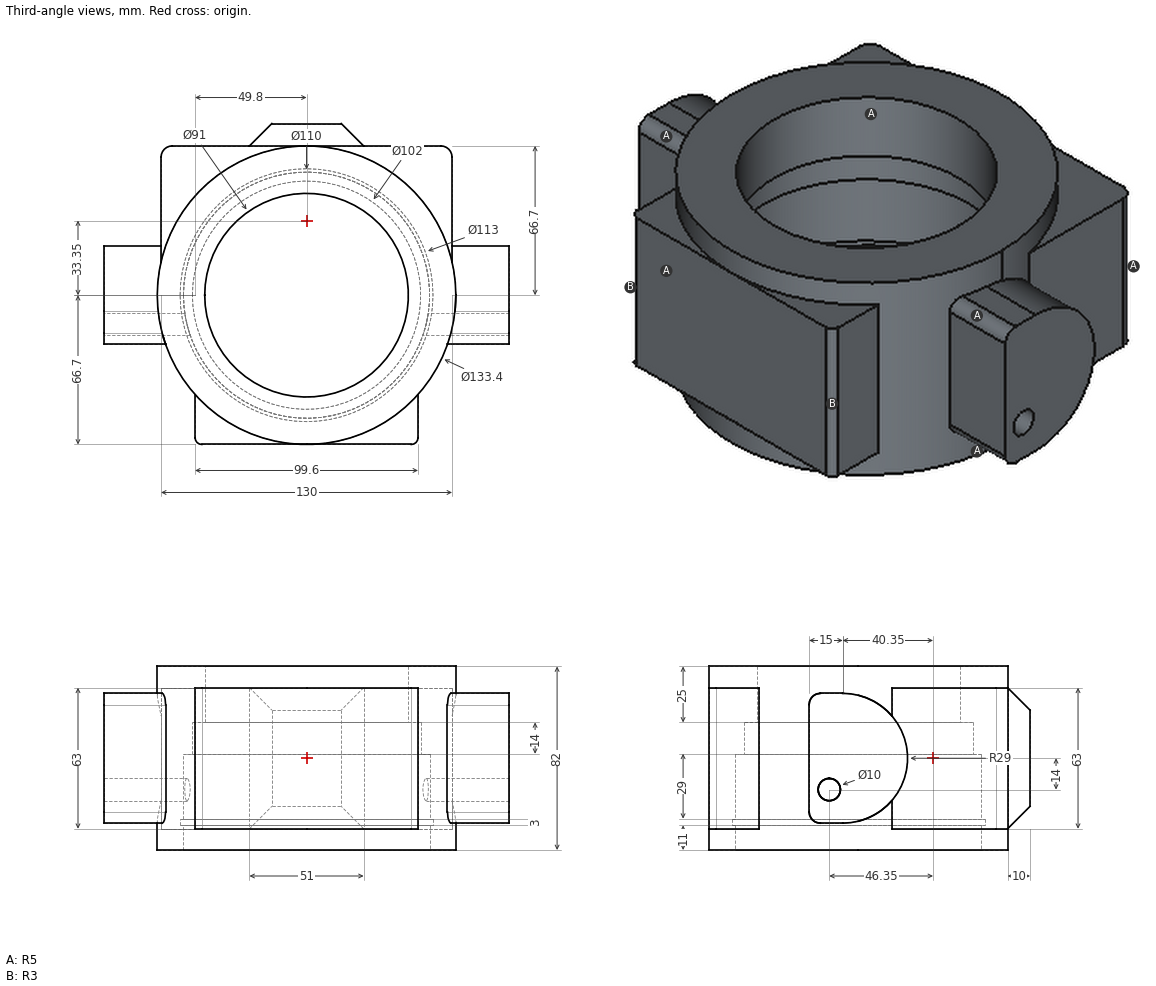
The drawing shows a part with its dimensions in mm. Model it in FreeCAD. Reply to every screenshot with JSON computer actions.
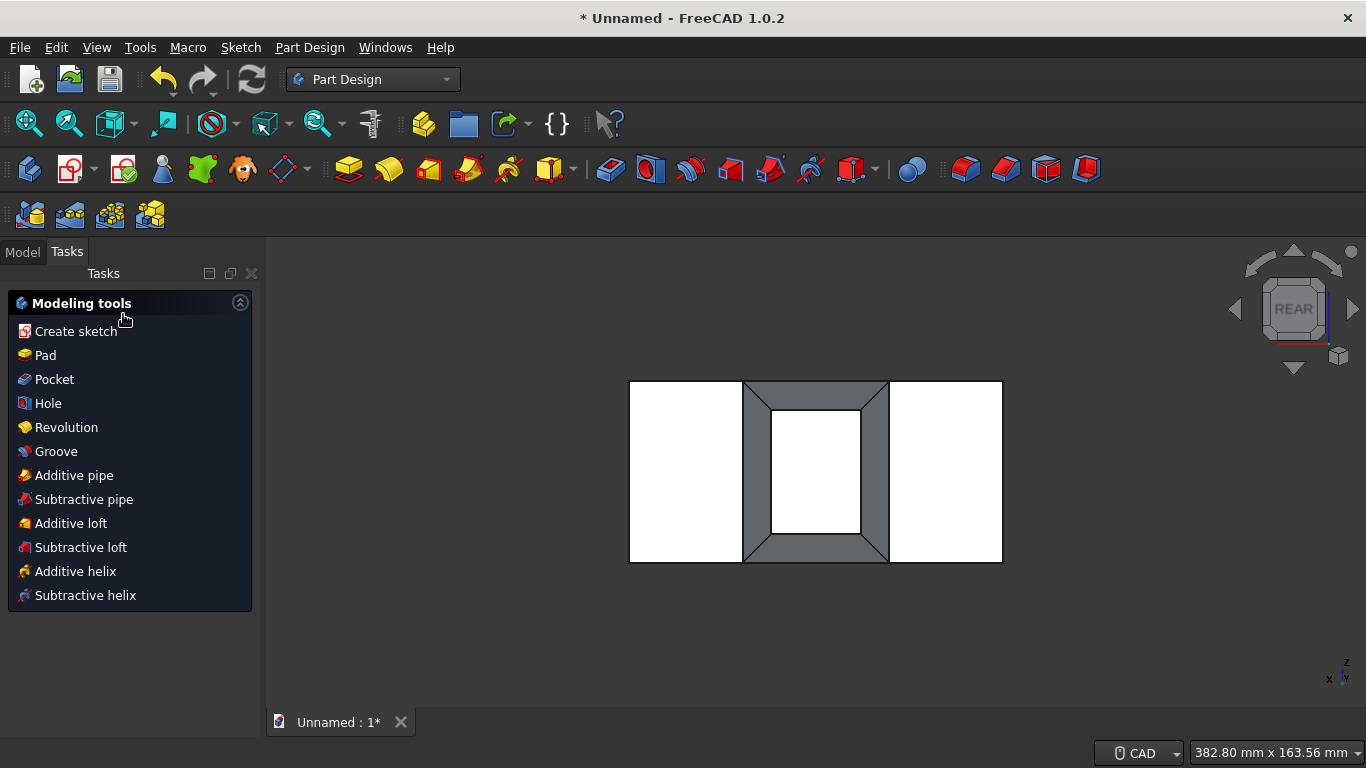
{"action": "left_click", "coordinate": [350, 170]}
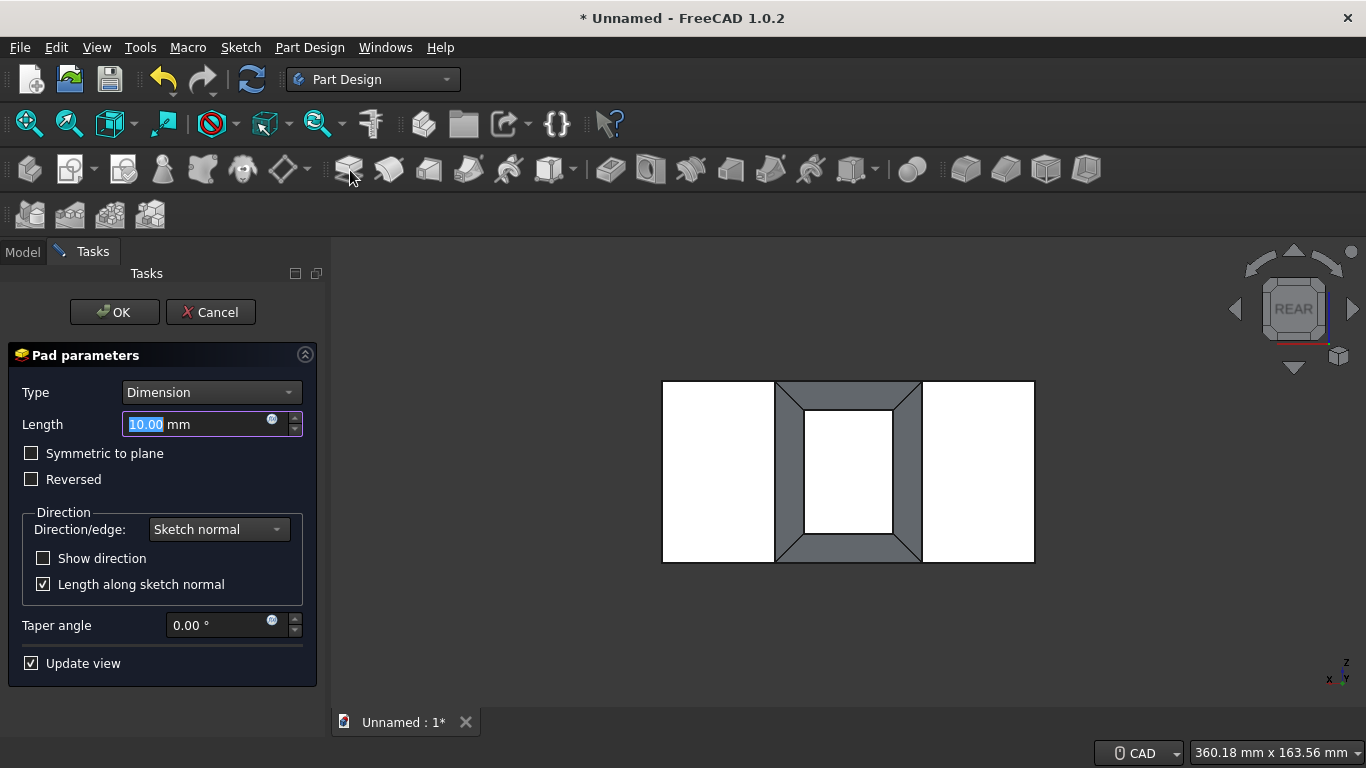
{"action": "type", "text": "63"}
{"action": "key", "text": "Tab"}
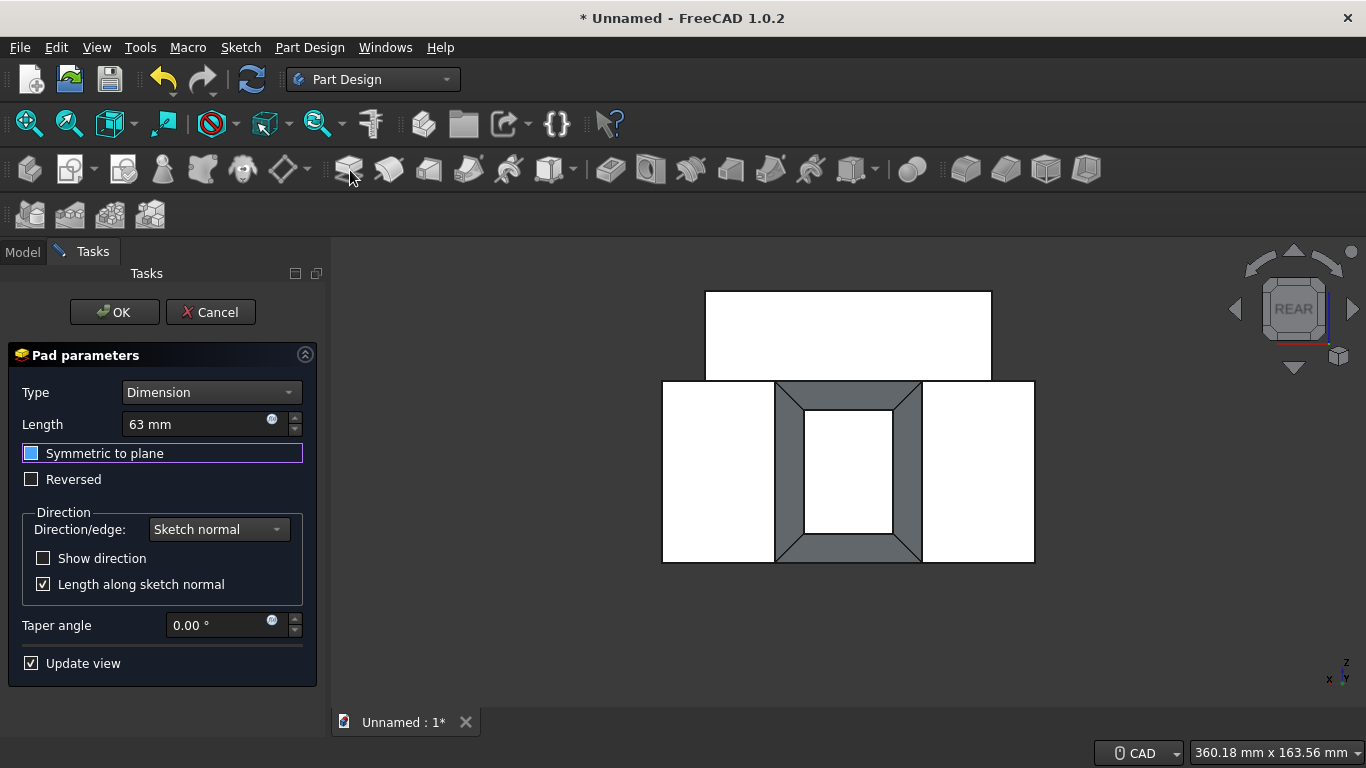
{"action": "left_click", "coordinate": [30, 453]}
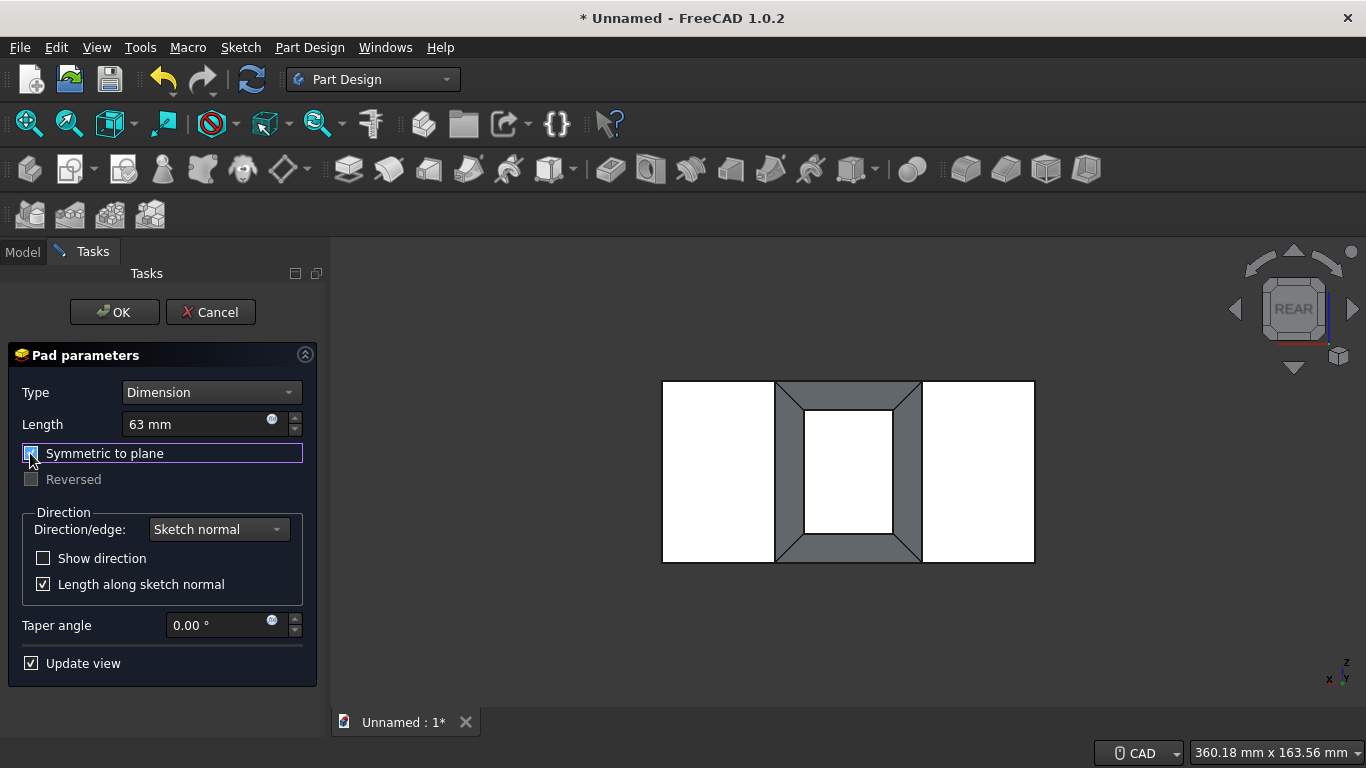
{"action": "left_click", "coordinate": [115, 312]}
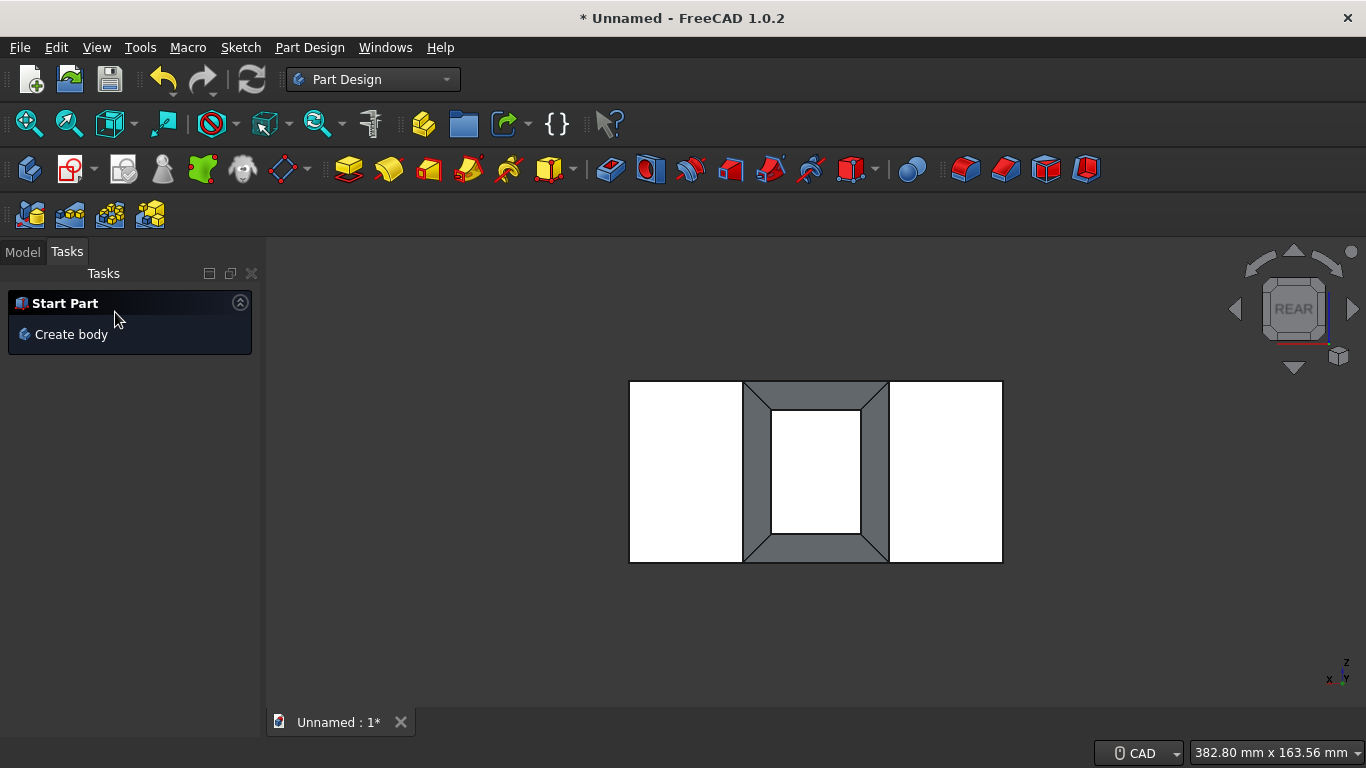
{"action": "key", "text": "v f"}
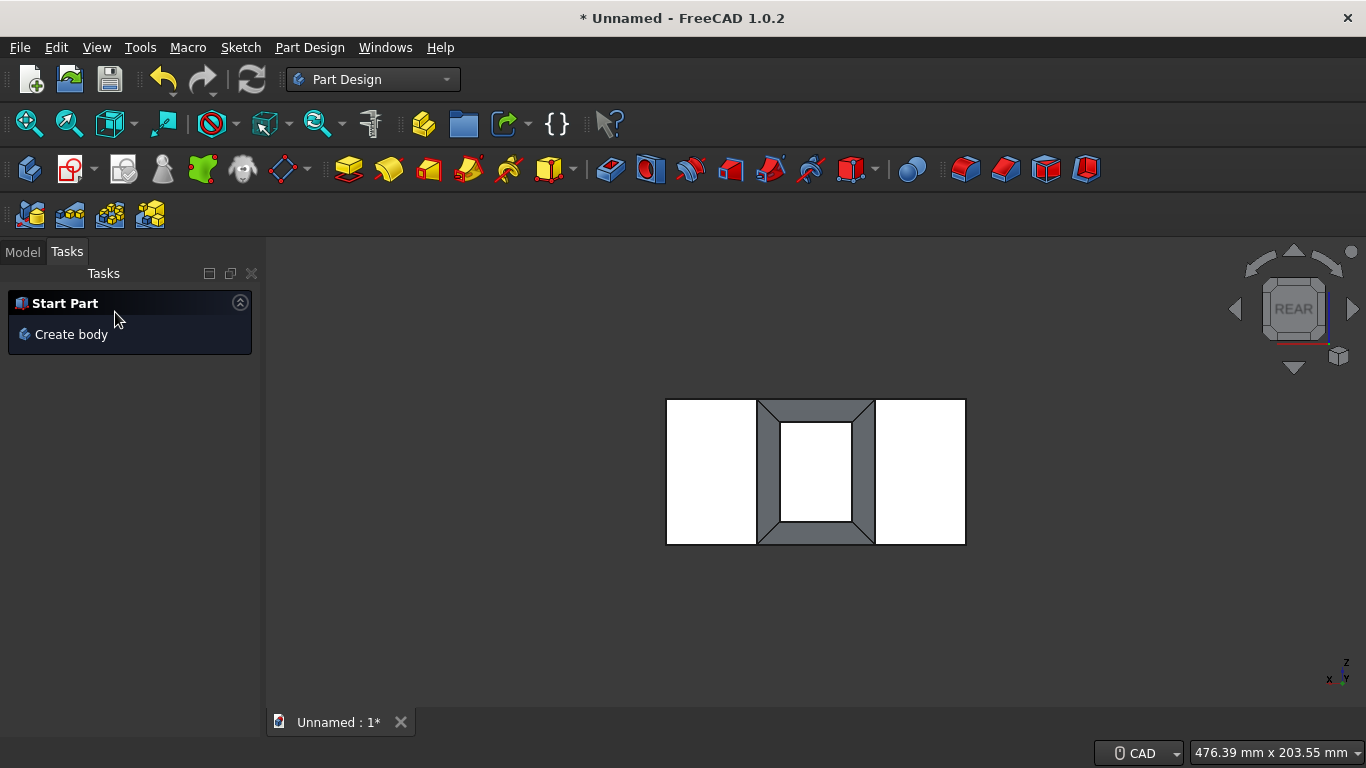
{"action": "left_click", "coordinate": [23, 251]}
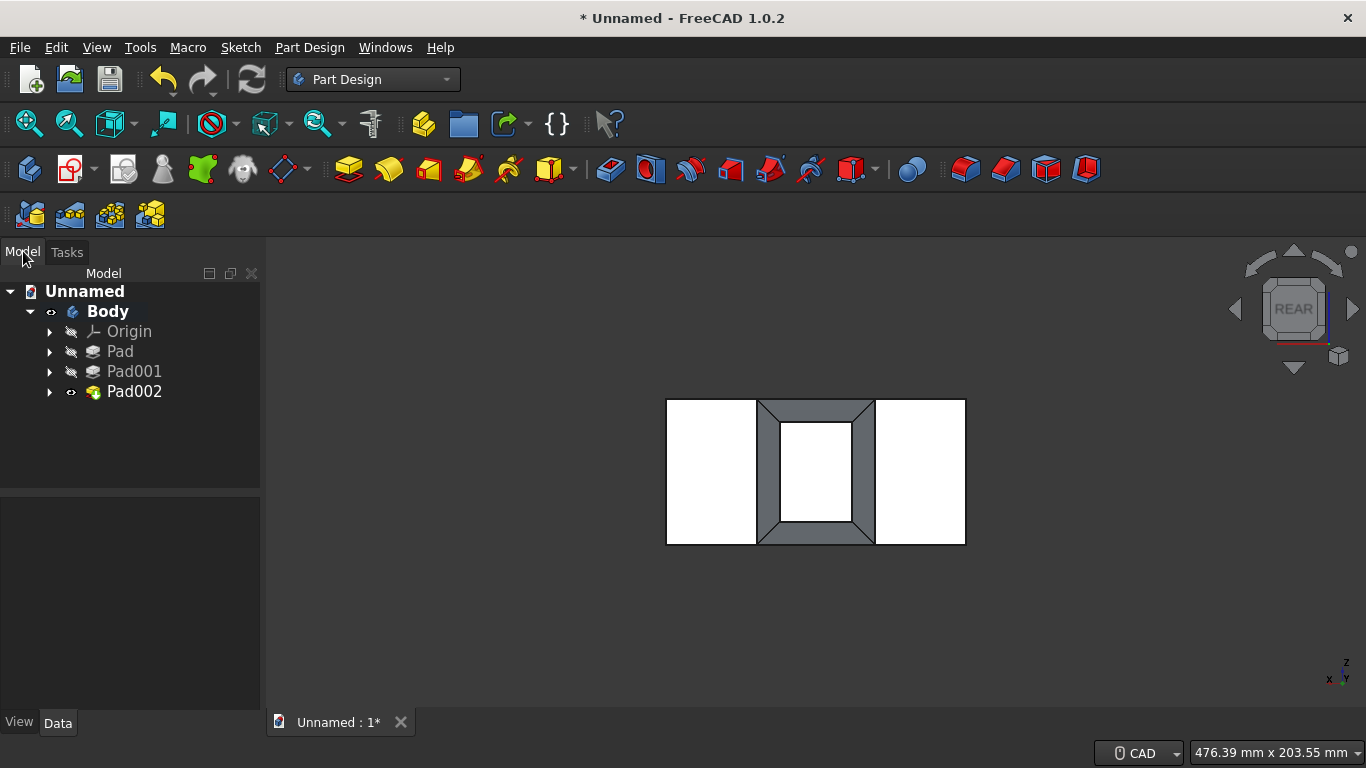
{"action": "left_click", "coordinate": [50, 332]}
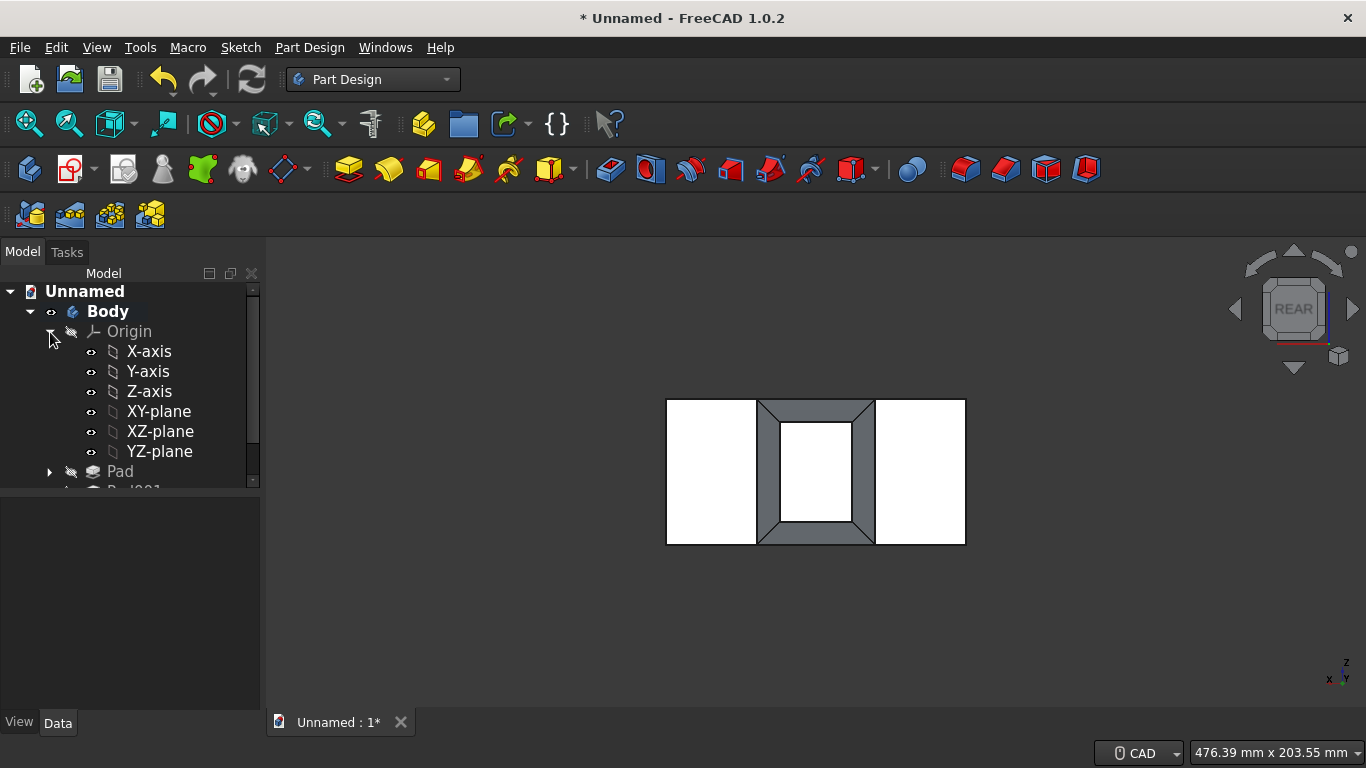
{"action": "left_click", "coordinate": [136, 412]}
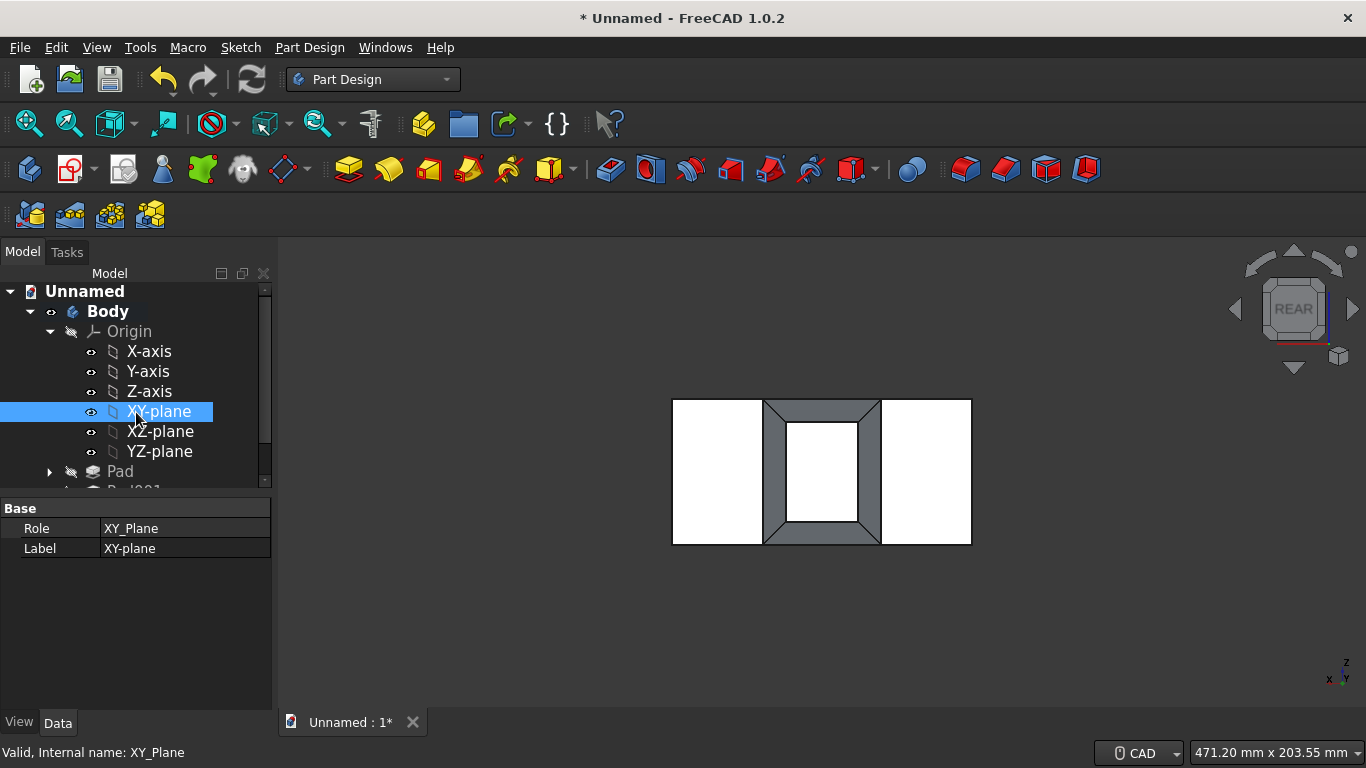
{"action": "left_click", "coordinate": [284, 170]}